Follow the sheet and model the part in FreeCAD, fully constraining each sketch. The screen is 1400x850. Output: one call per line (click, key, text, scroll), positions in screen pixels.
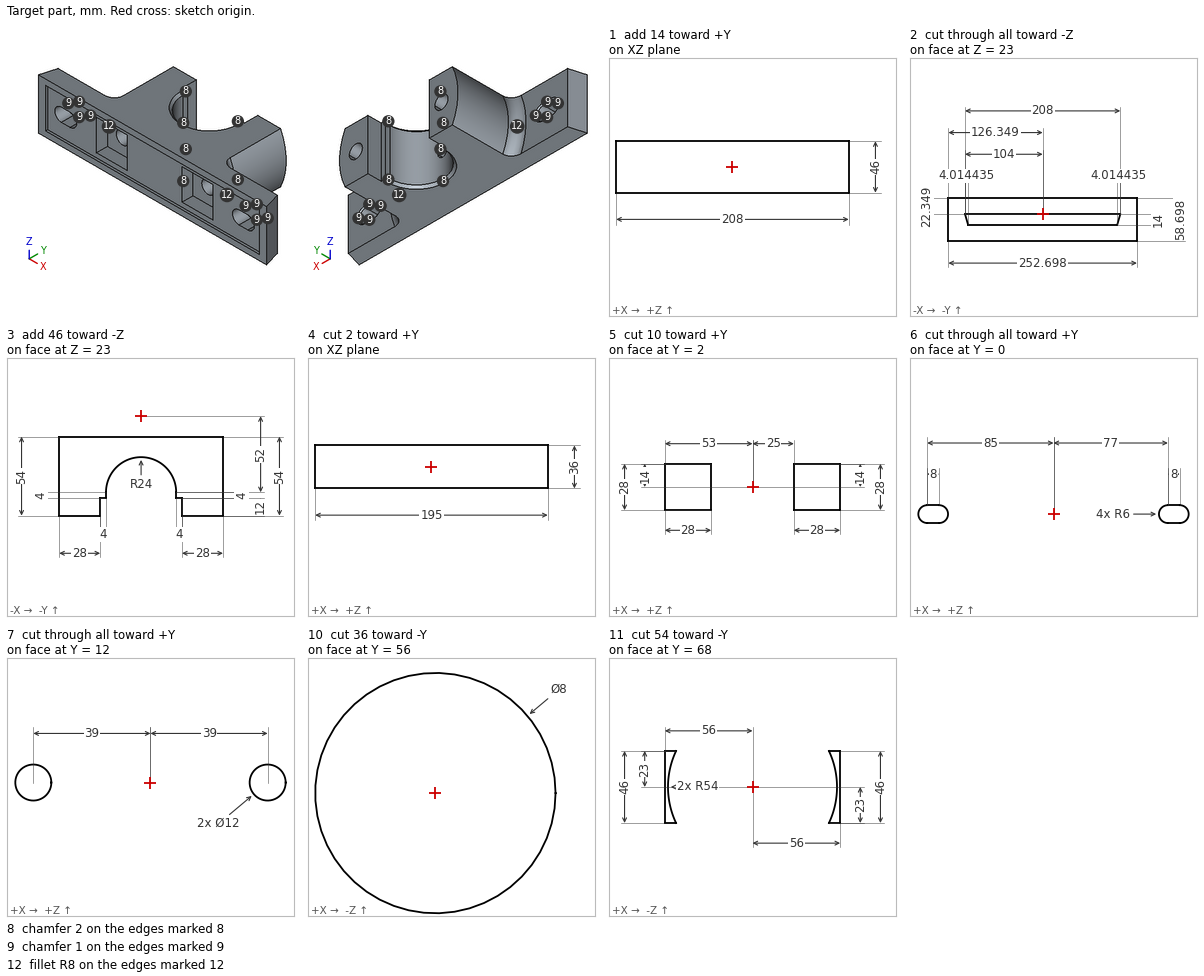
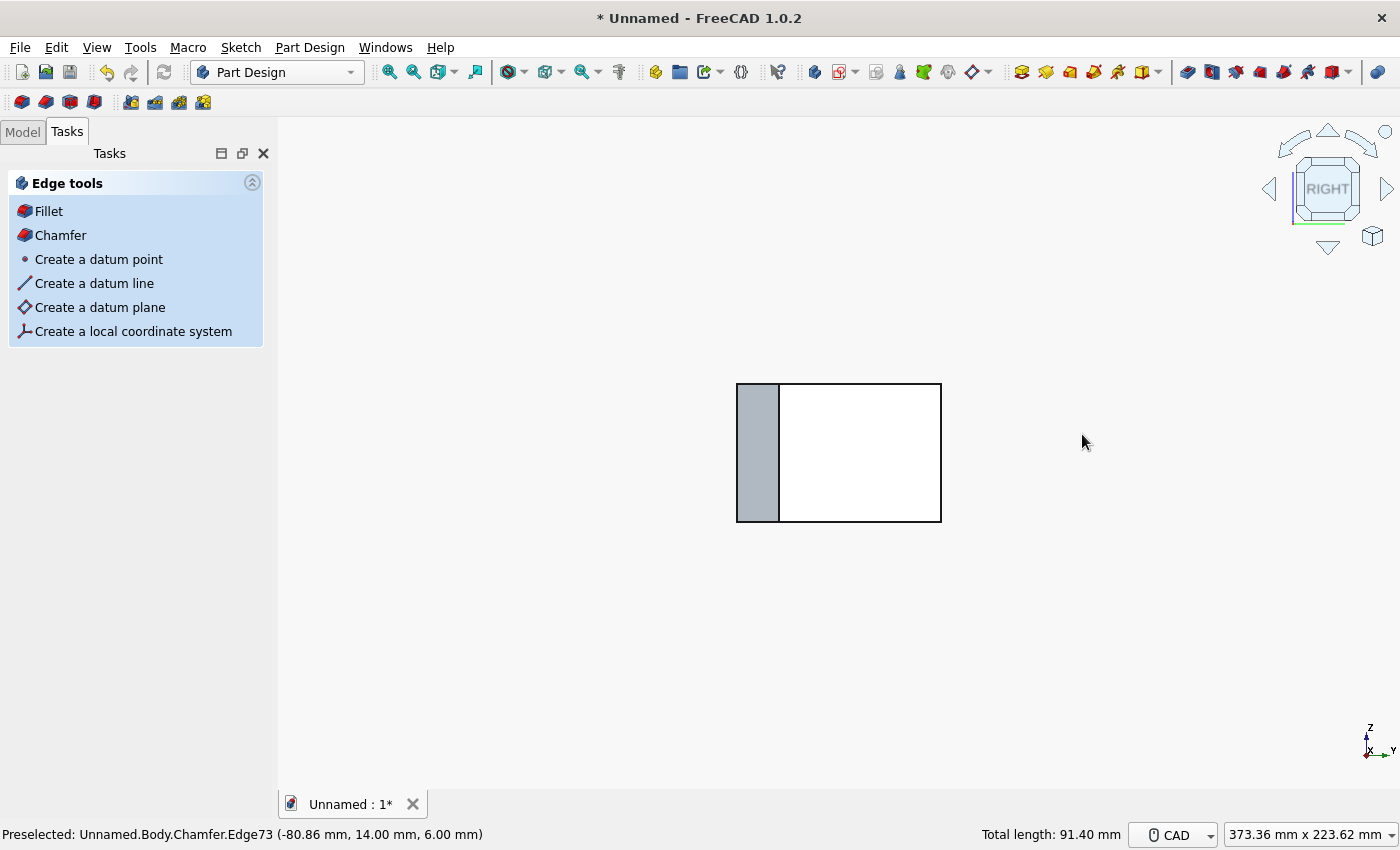
key(v)
key(f)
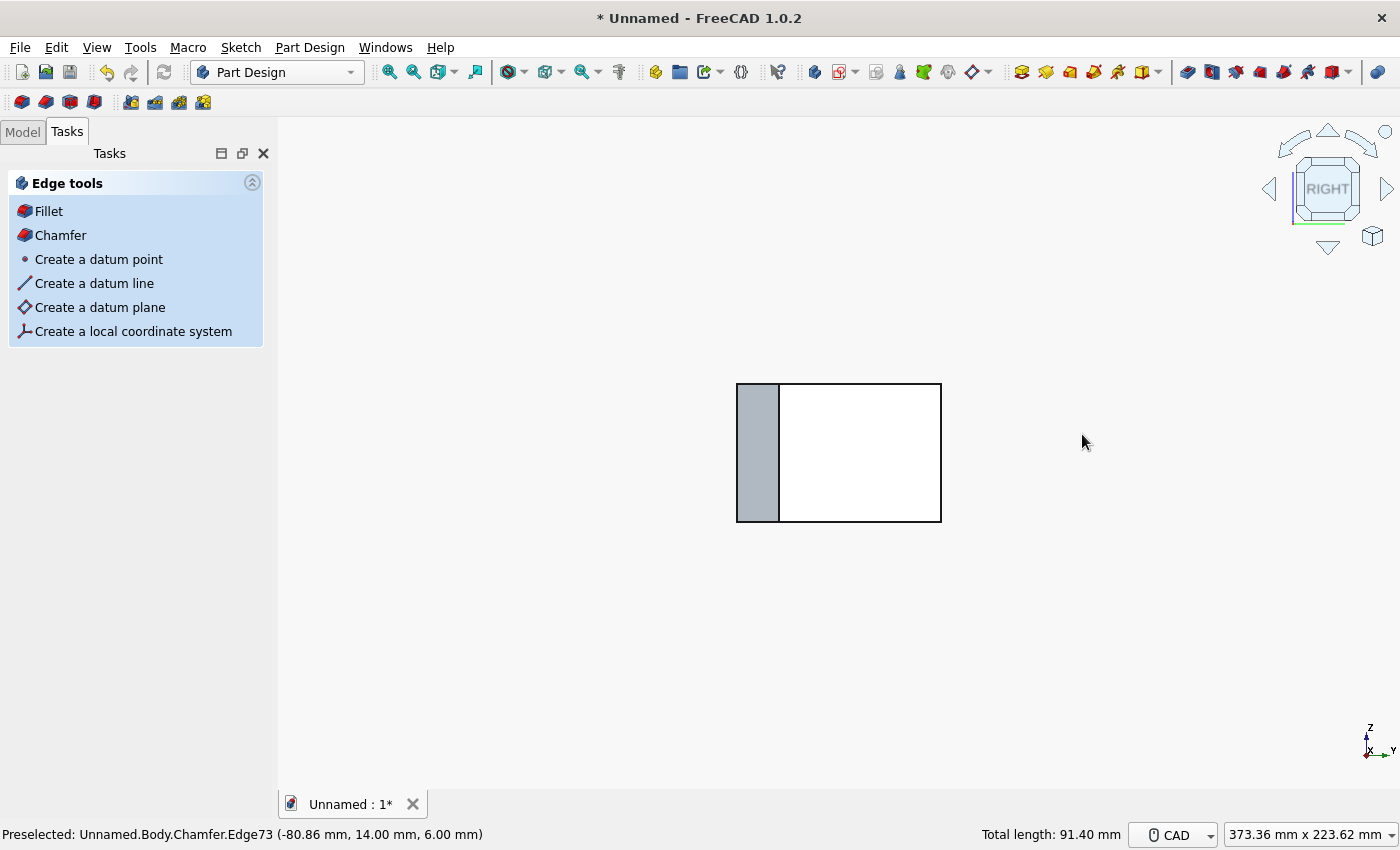
key(5)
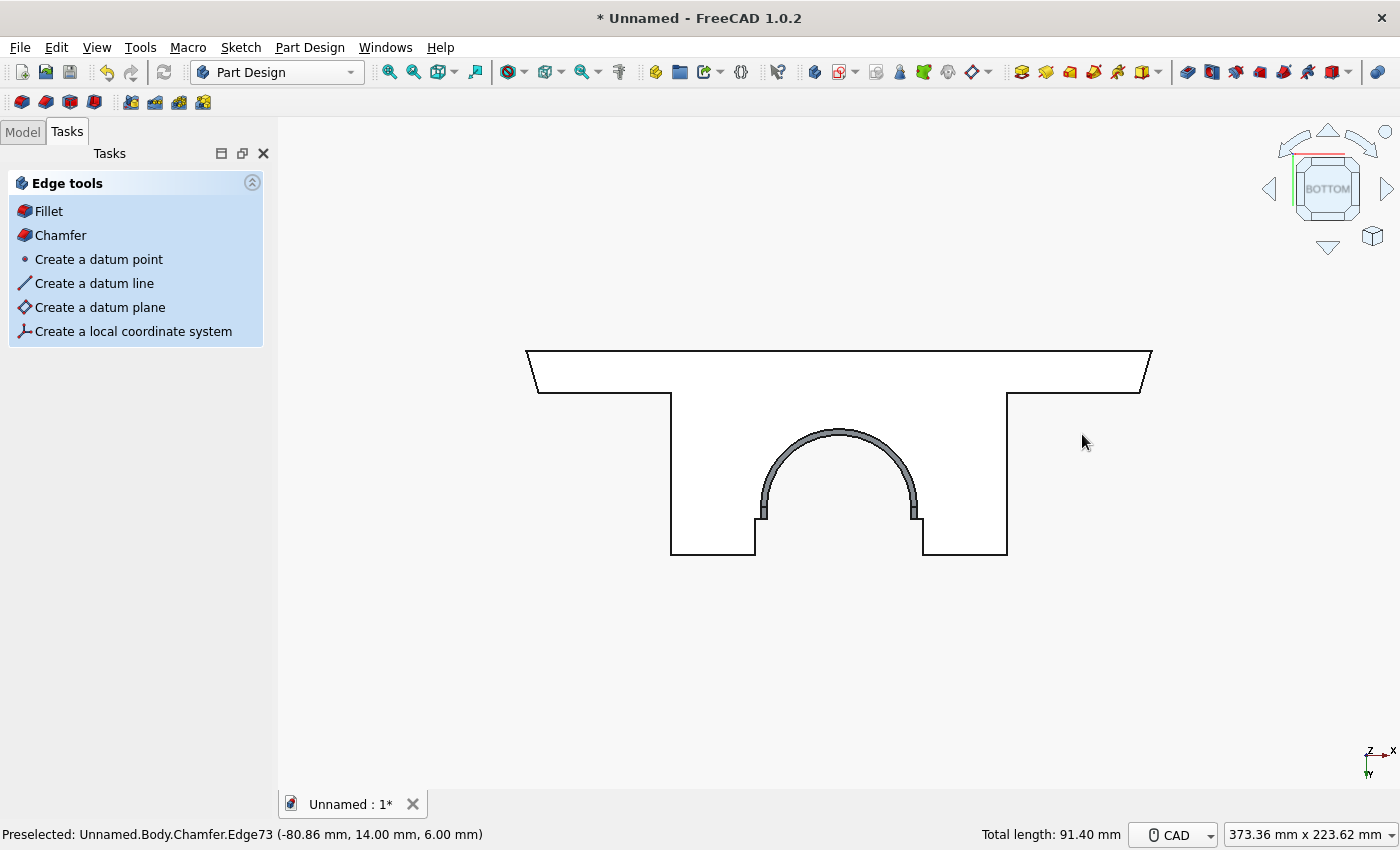
key(4)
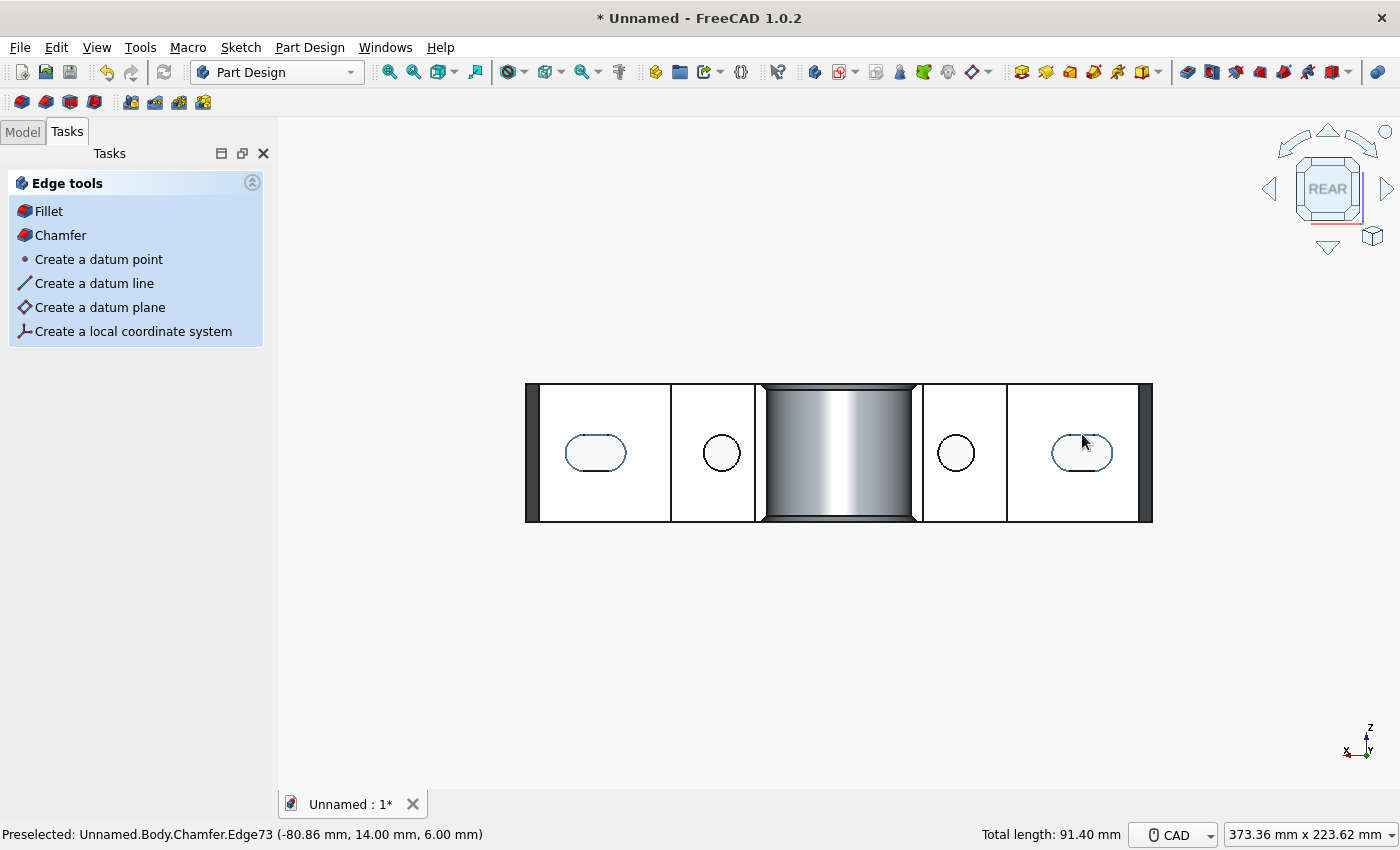
key(6)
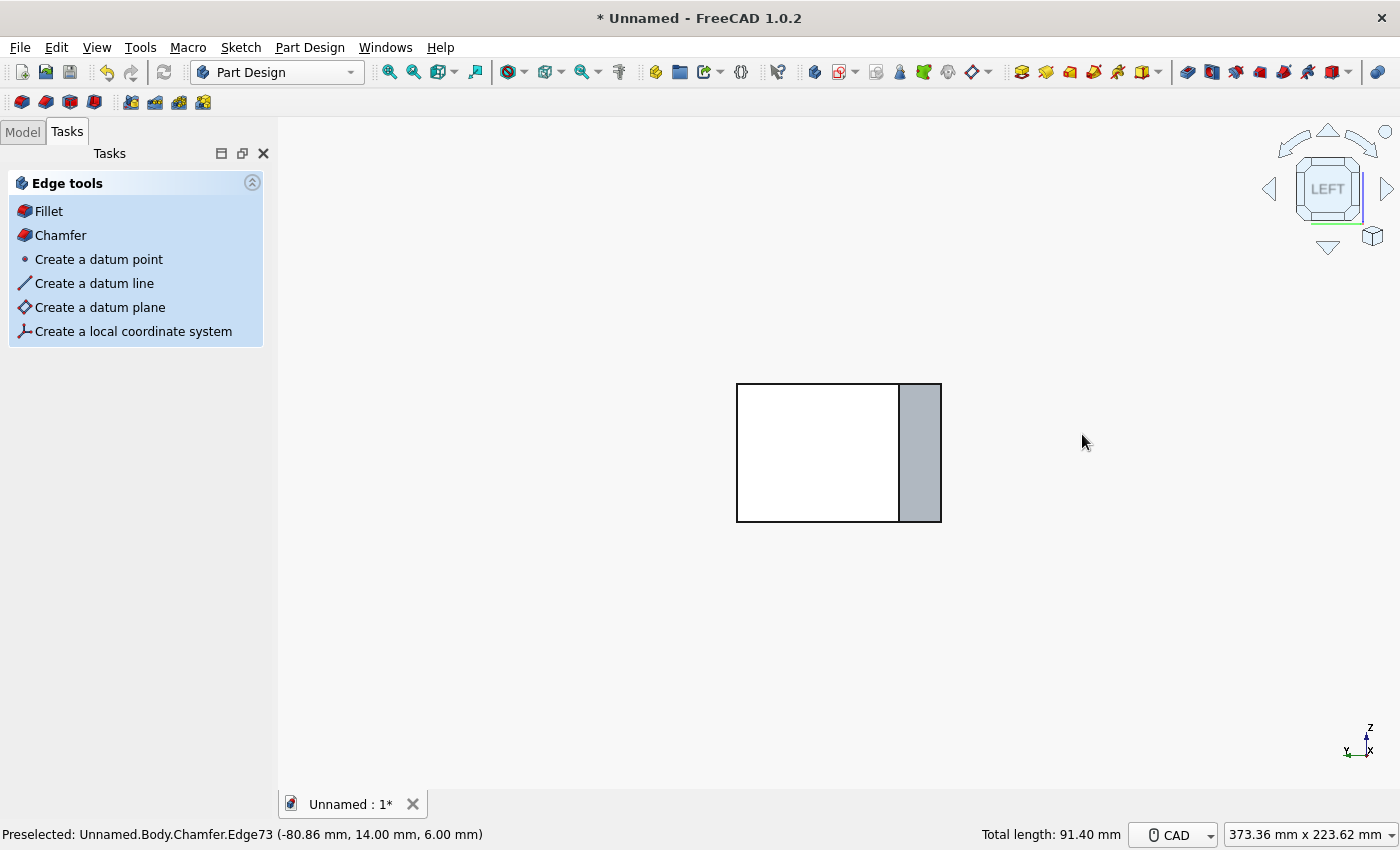
key(v)
key(f)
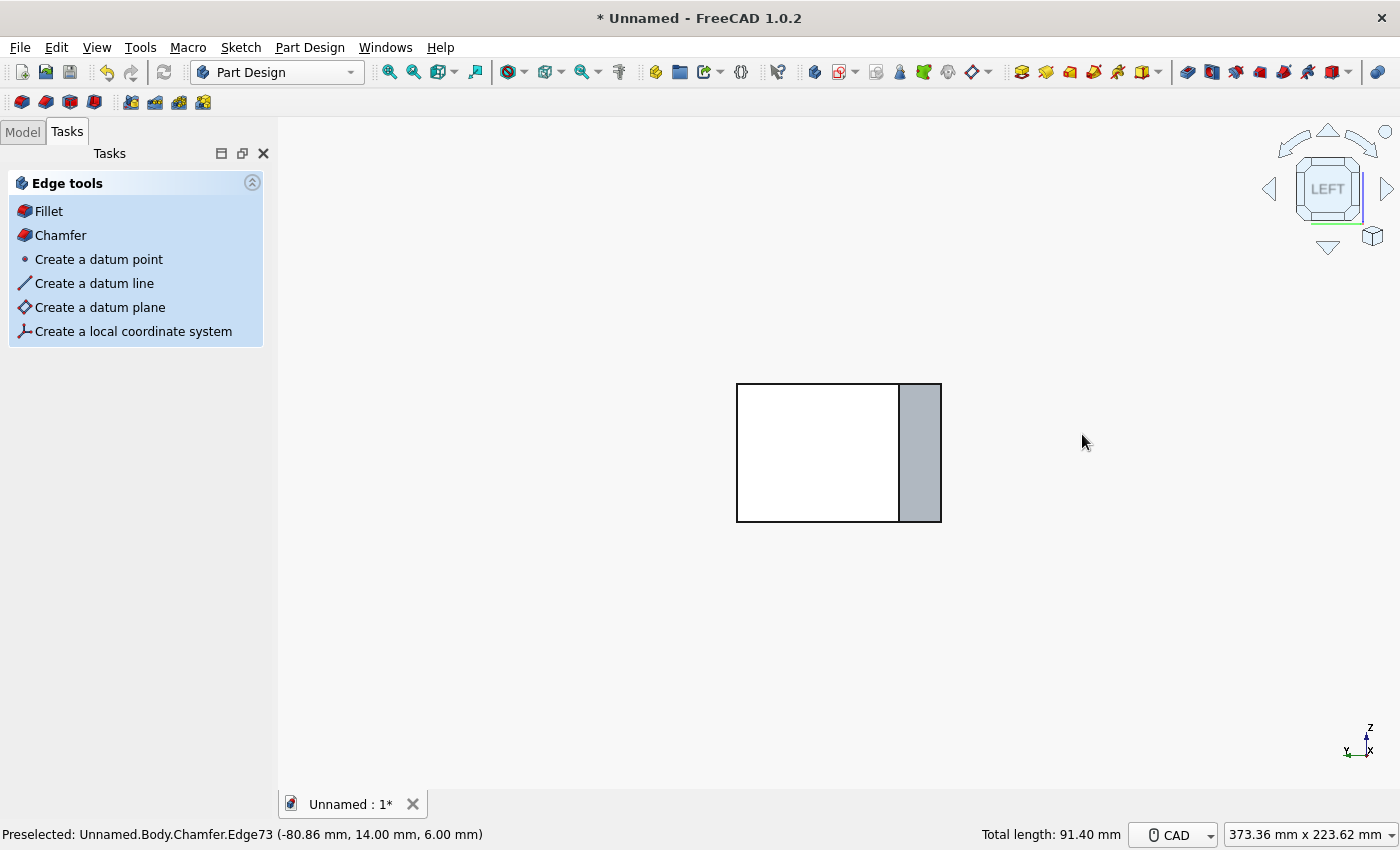
key(v)
key(3)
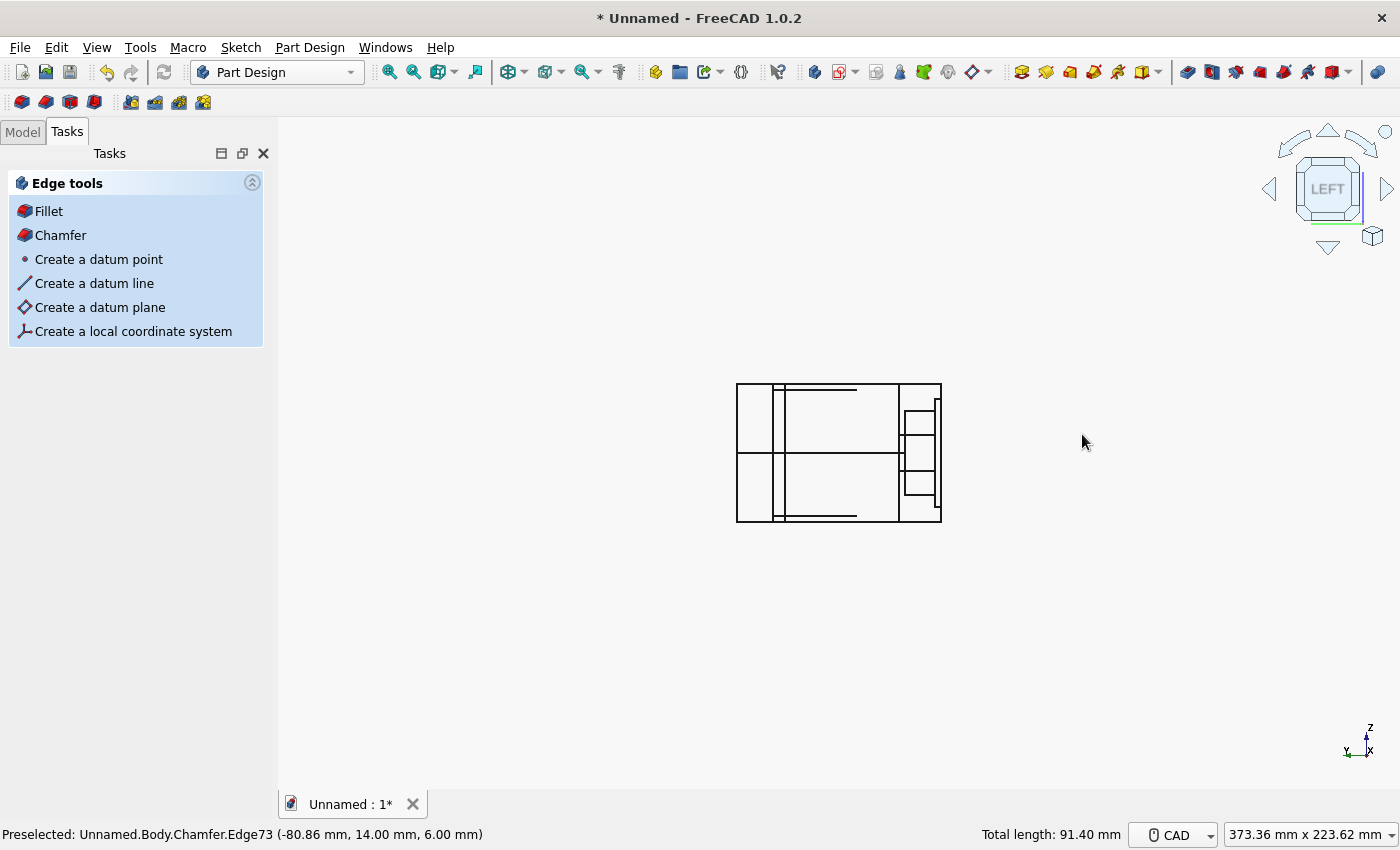
key(0)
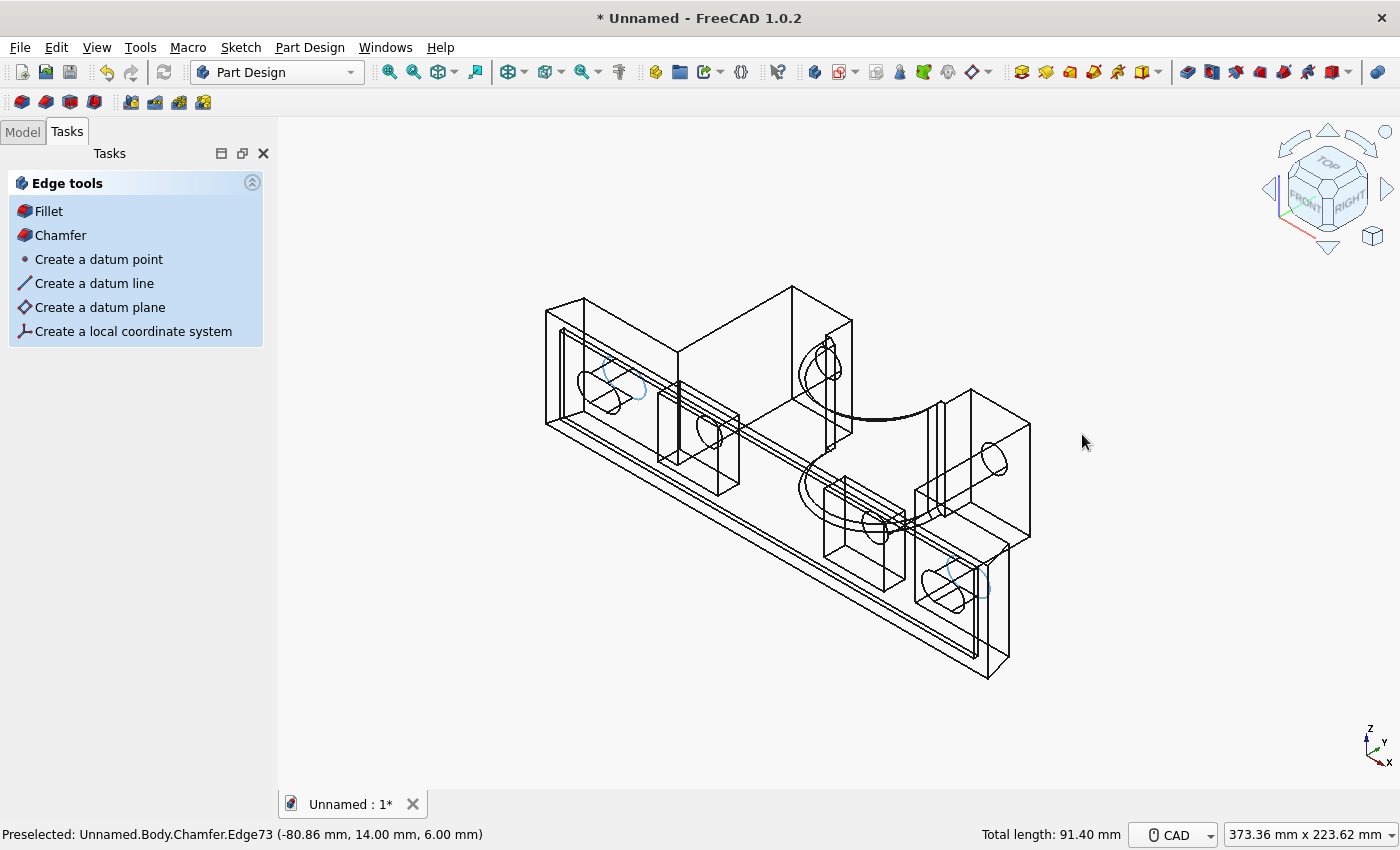
click(624, 392, ctrl)